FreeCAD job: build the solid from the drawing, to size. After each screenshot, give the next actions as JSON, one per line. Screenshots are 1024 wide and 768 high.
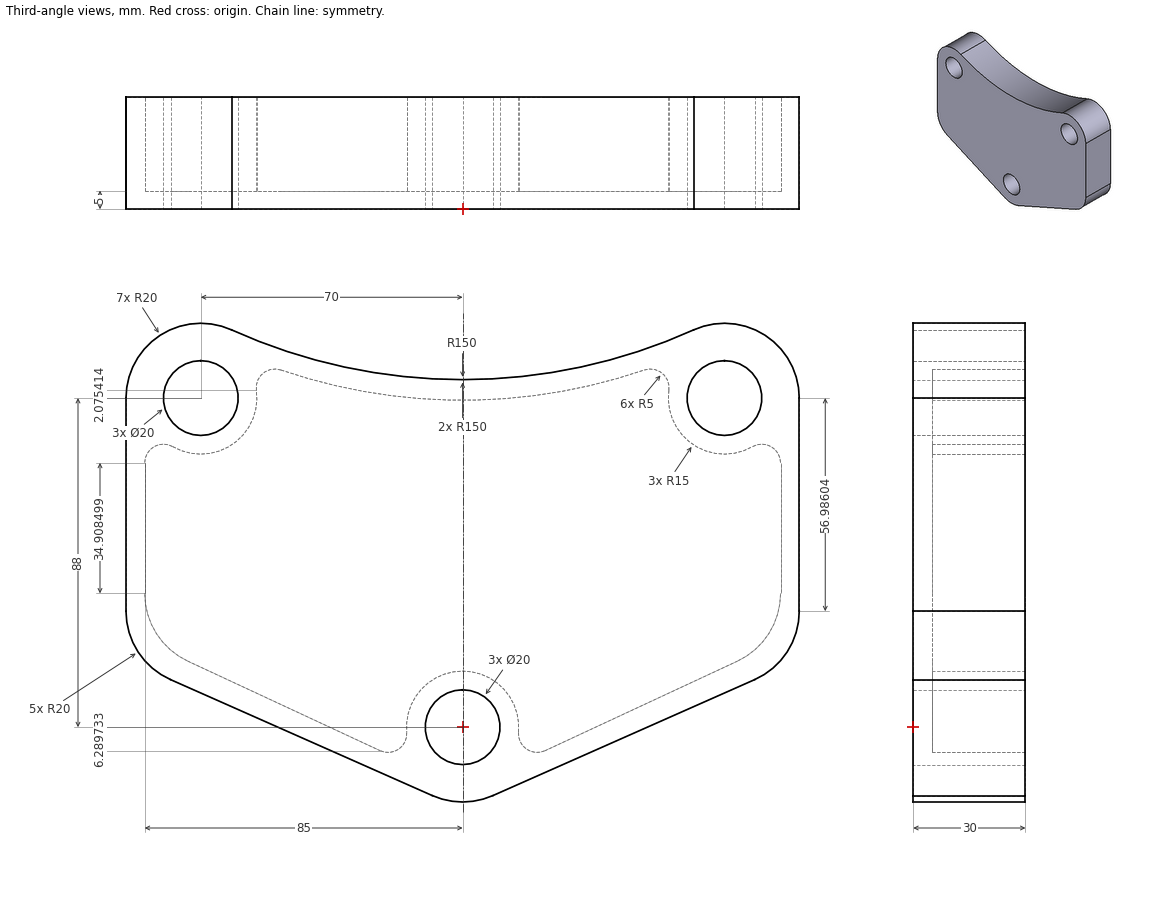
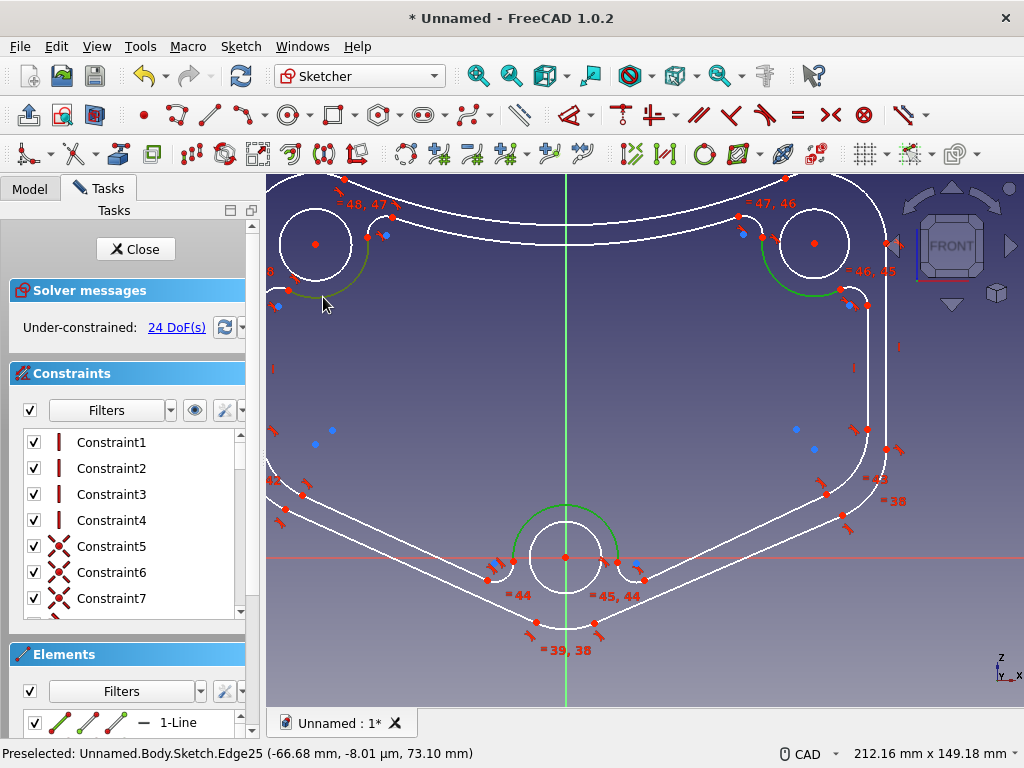
{"action": "left_click", "coordinate": [798, 116]}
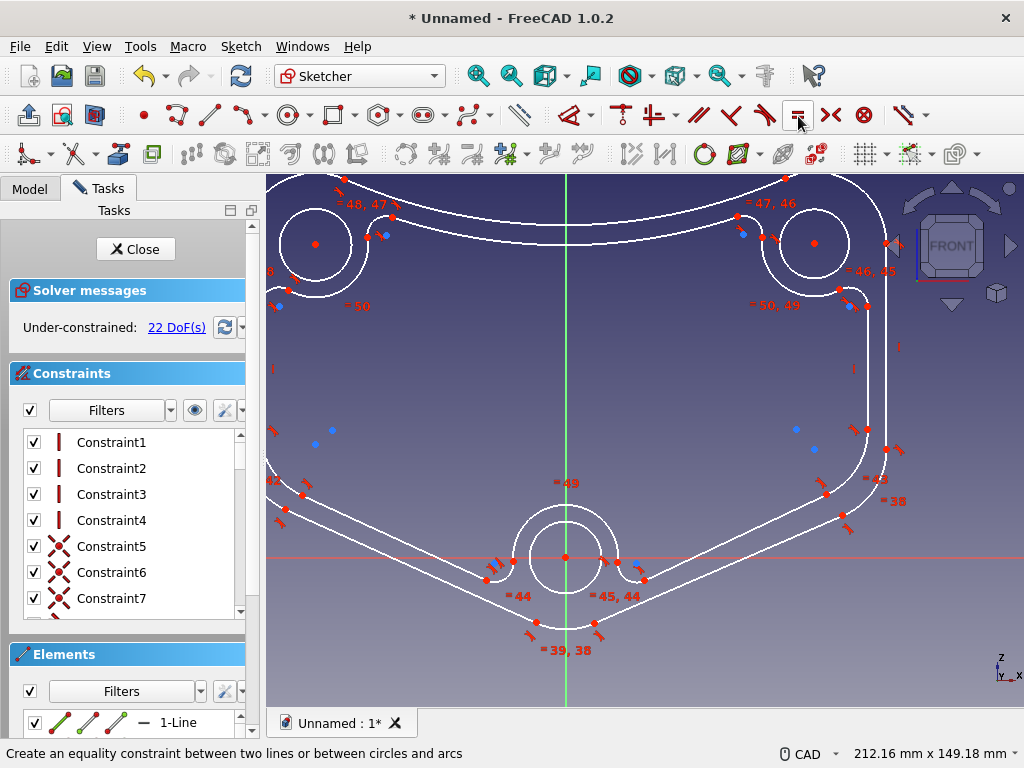
{"action": "left_click", "coordinate": [475, 218]}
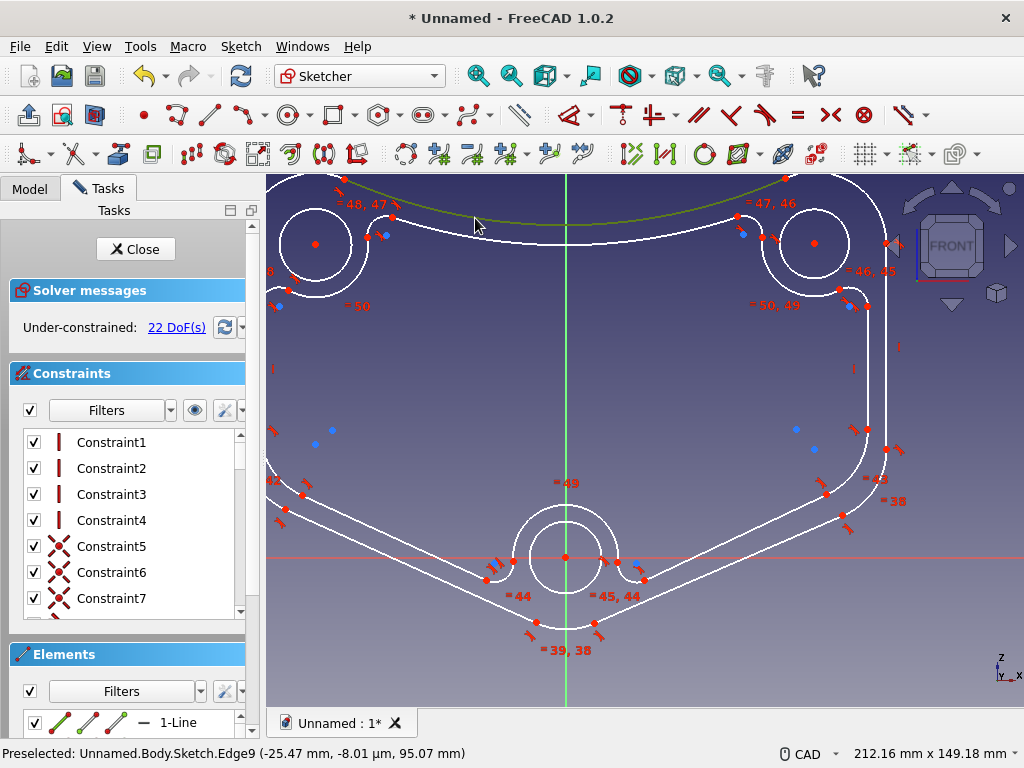
{"action": "left_click", "coordinate": [495, 241]}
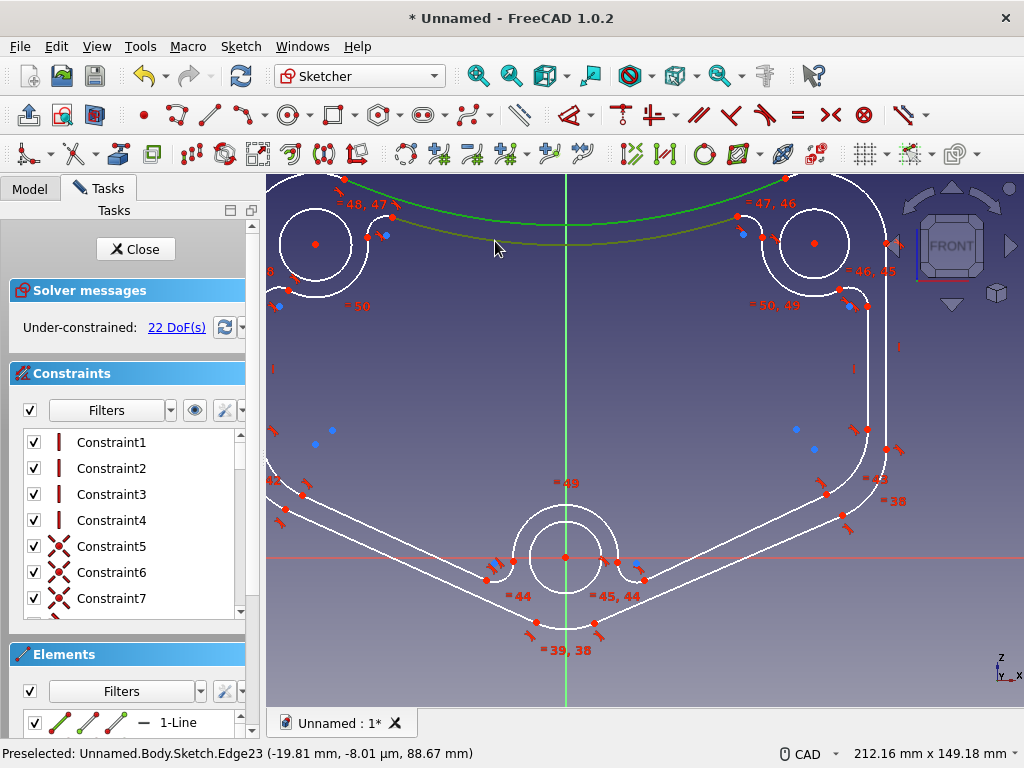
{"action": "left_click", "coordinate": [798, 116]}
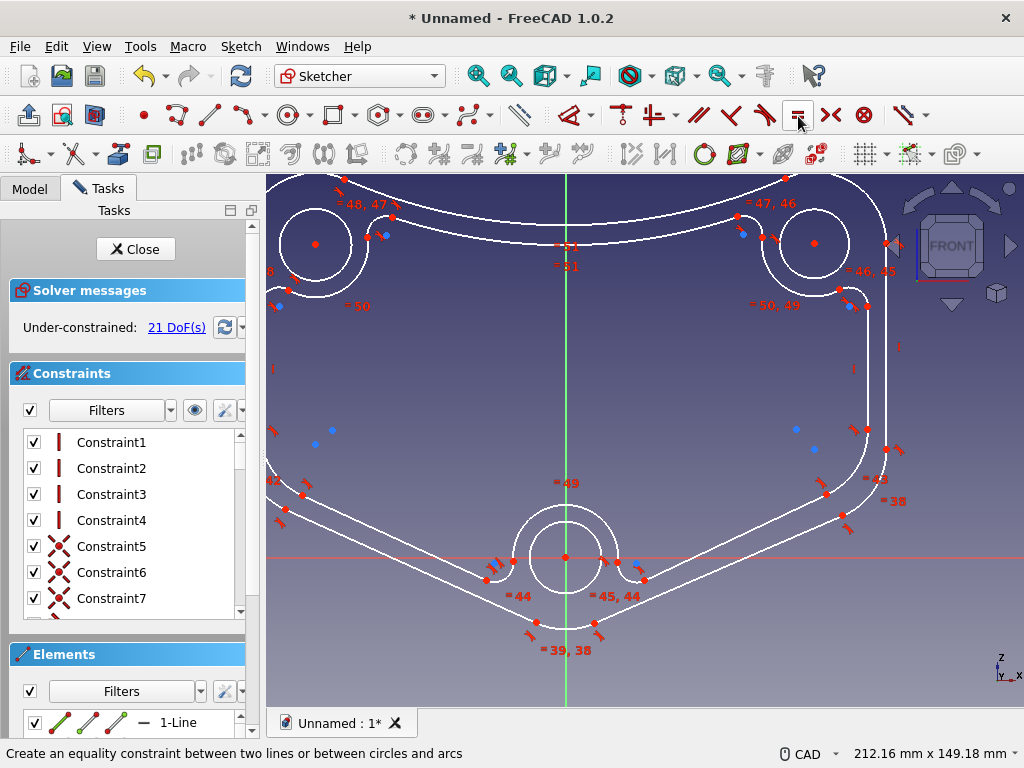
{"action": "left_click", "coordinate": [341, 219]}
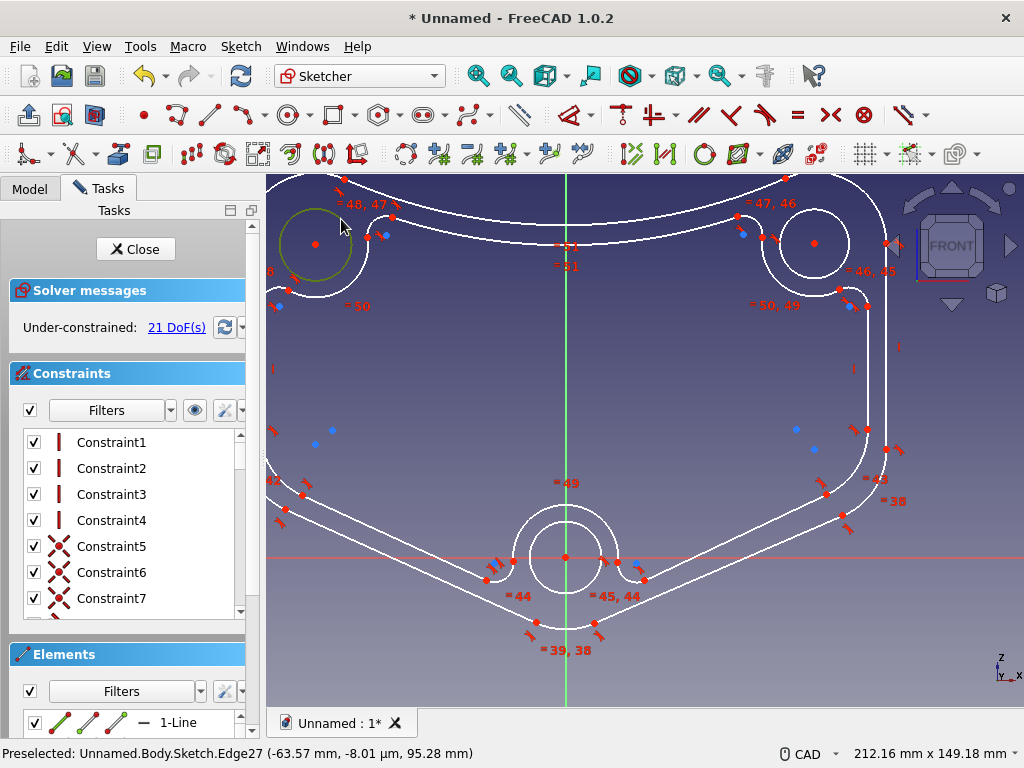
{"action": "left_click", "coordinate": [839, 219]}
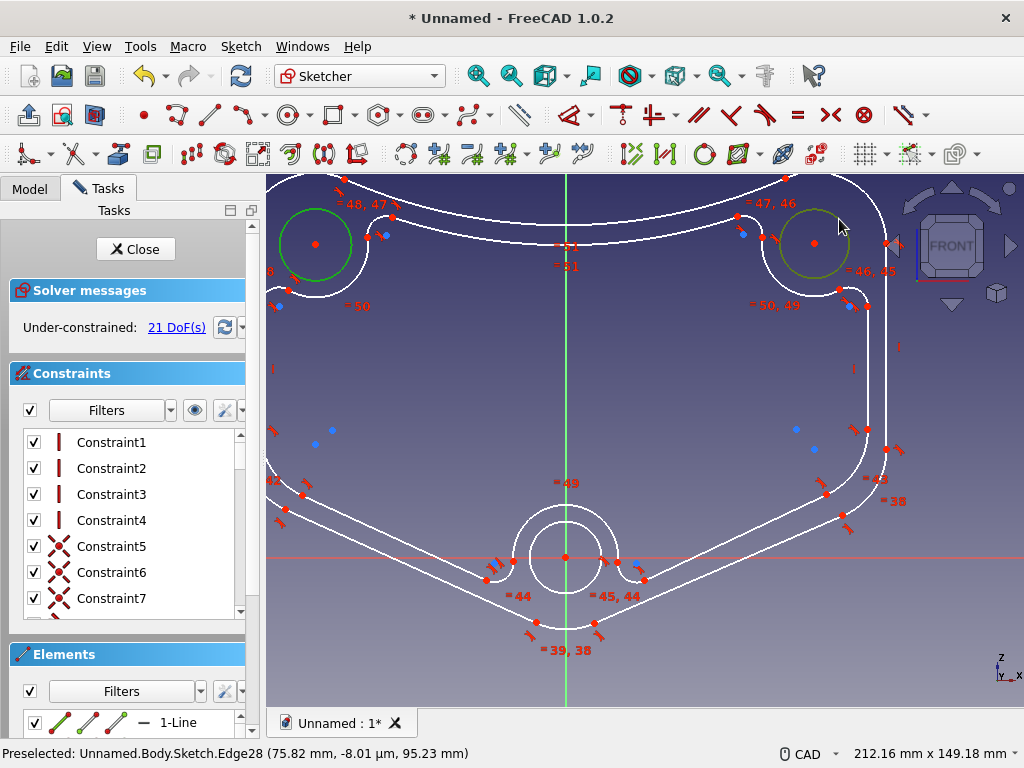
{"action": "left_click", "coordinate": [591, 532]}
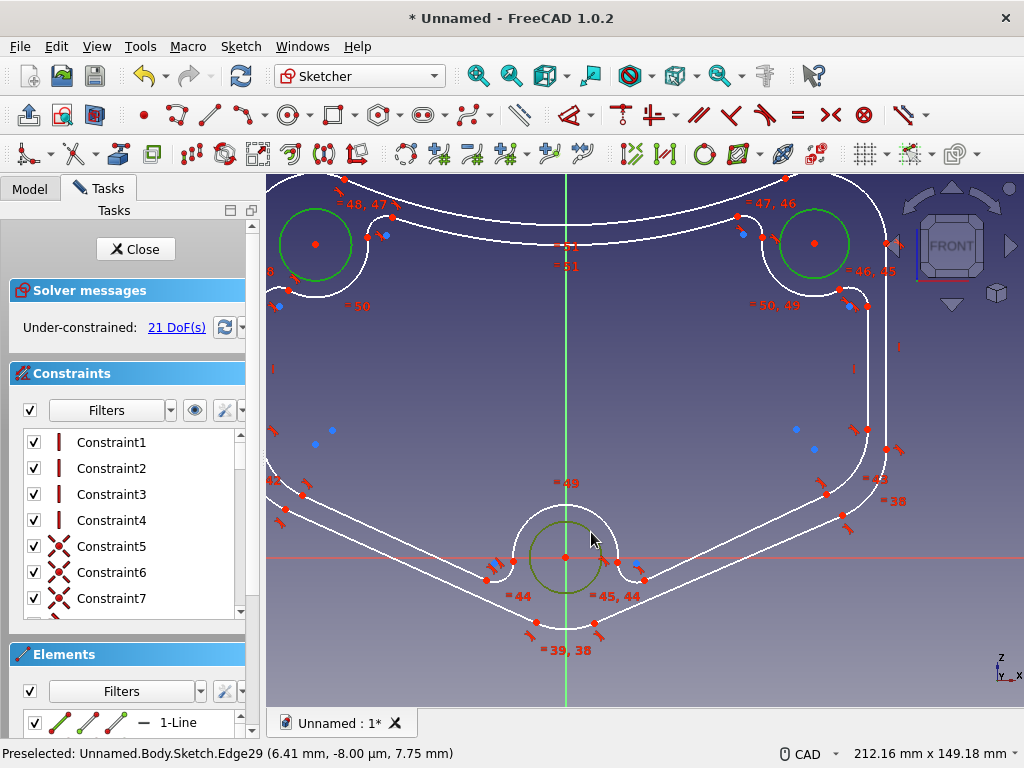
{"action": "left_click", "coordinate": [798, 116]}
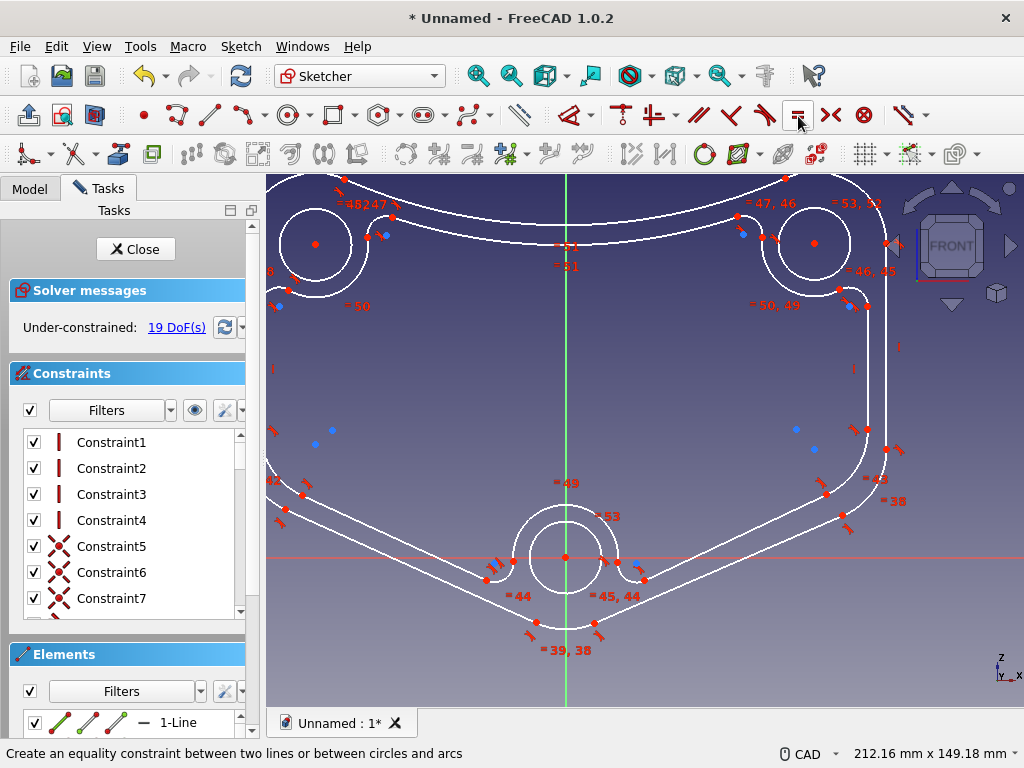
{"action": "scroll", "coordinate": [599, 516], "scroll_direction": "down", "scroll_amount": 2}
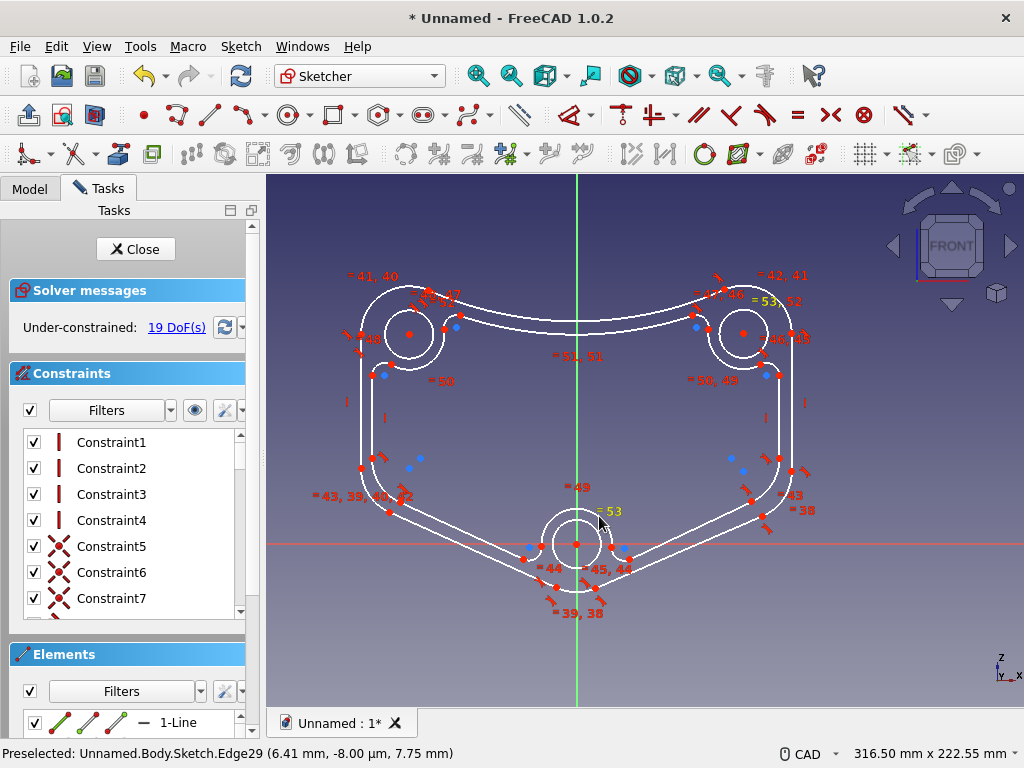
{"action": "scroll", "coordinate": [576, 643], "scroll_direction": "down", "scroll_amount": 3}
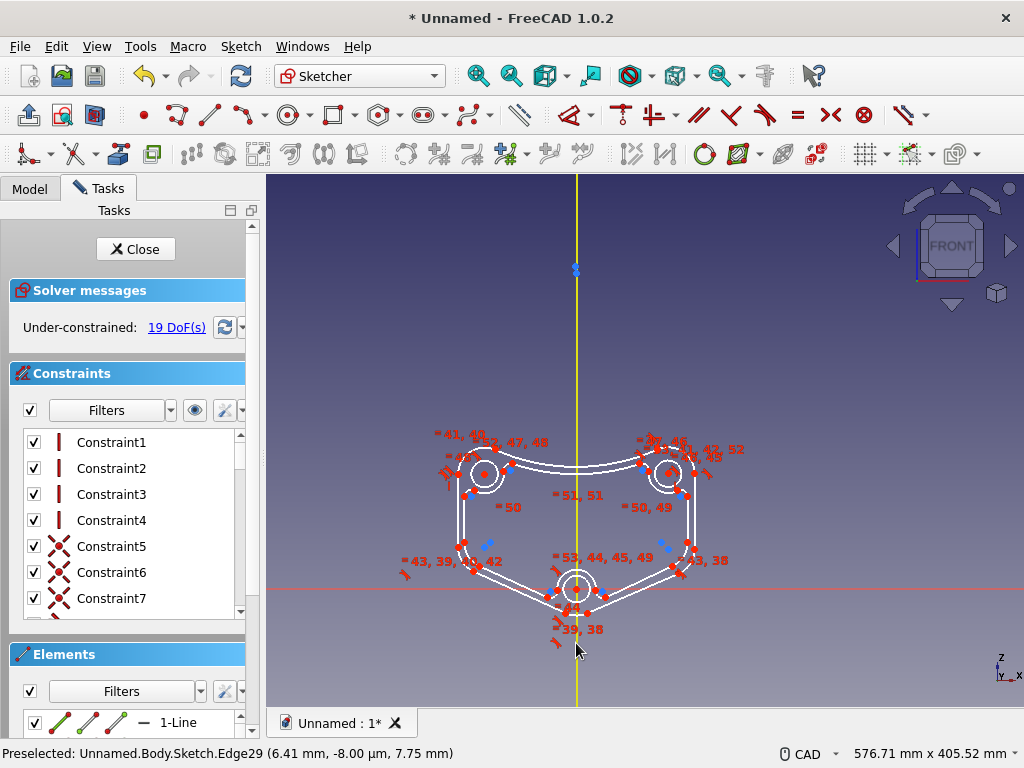
{"action": "scroll", "coordinate": [576, 266], "scroll_direction": "up", "scroll_amount": 3}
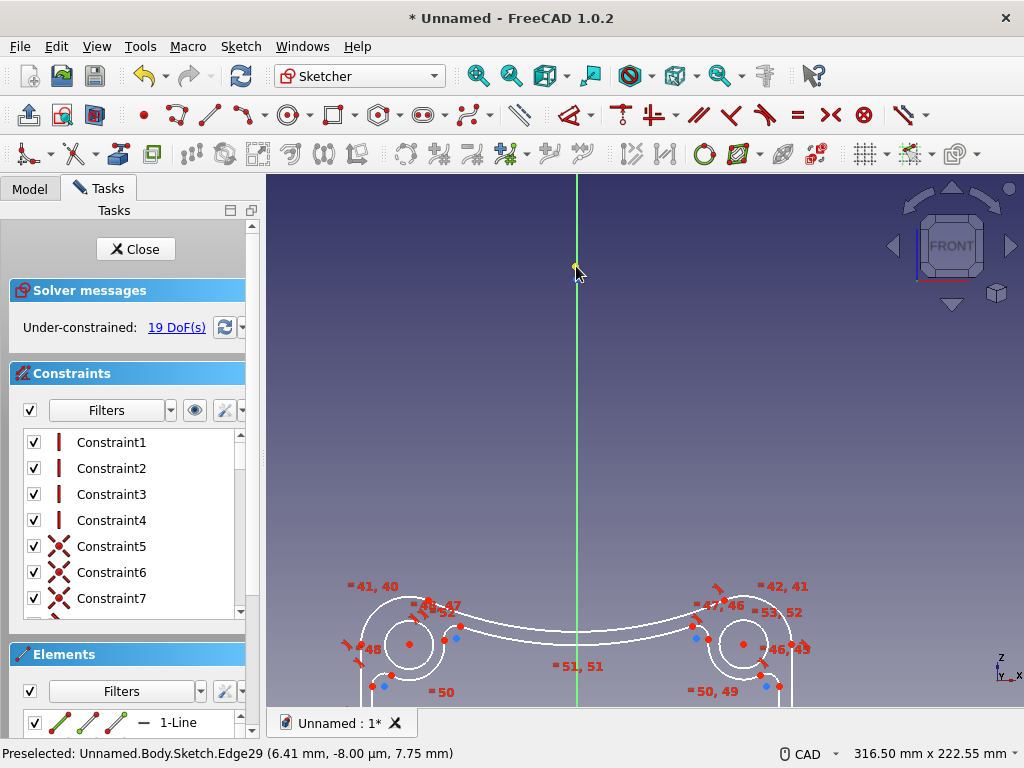
{"action": "left_click", "coordinate": [576, 266]}